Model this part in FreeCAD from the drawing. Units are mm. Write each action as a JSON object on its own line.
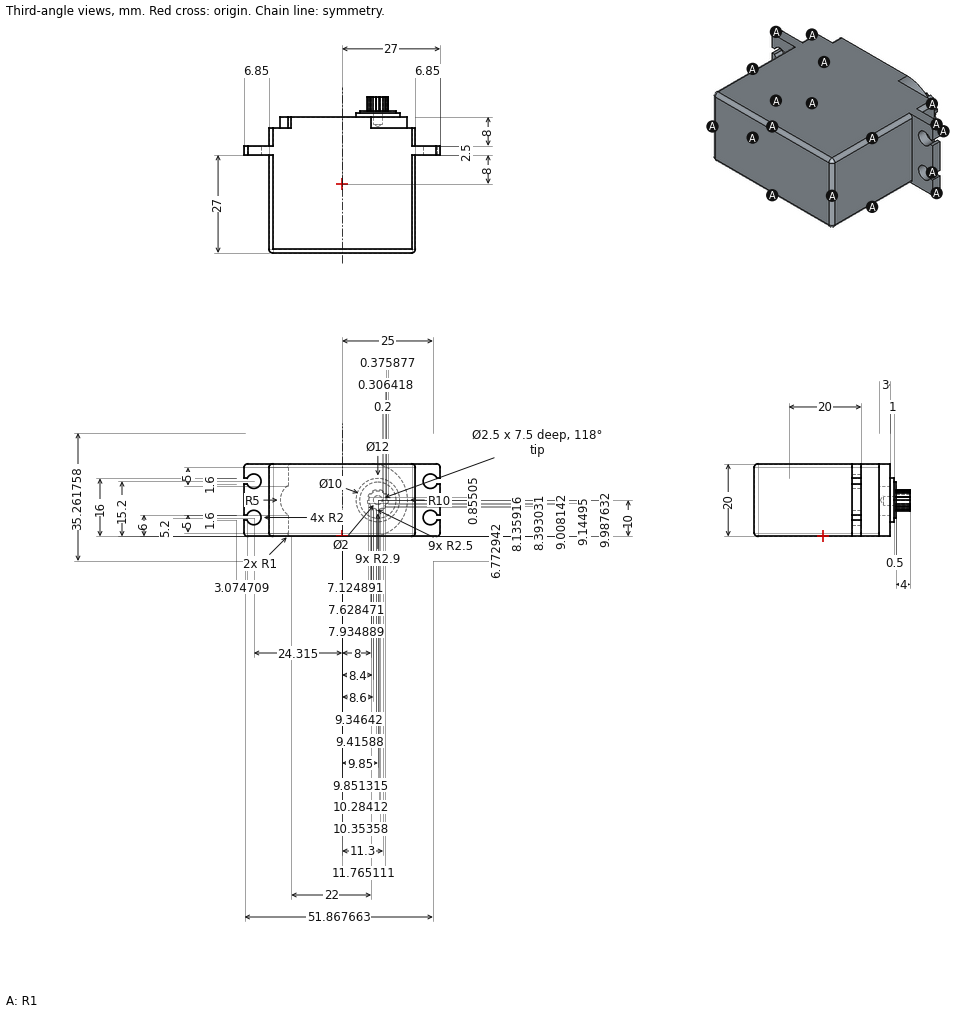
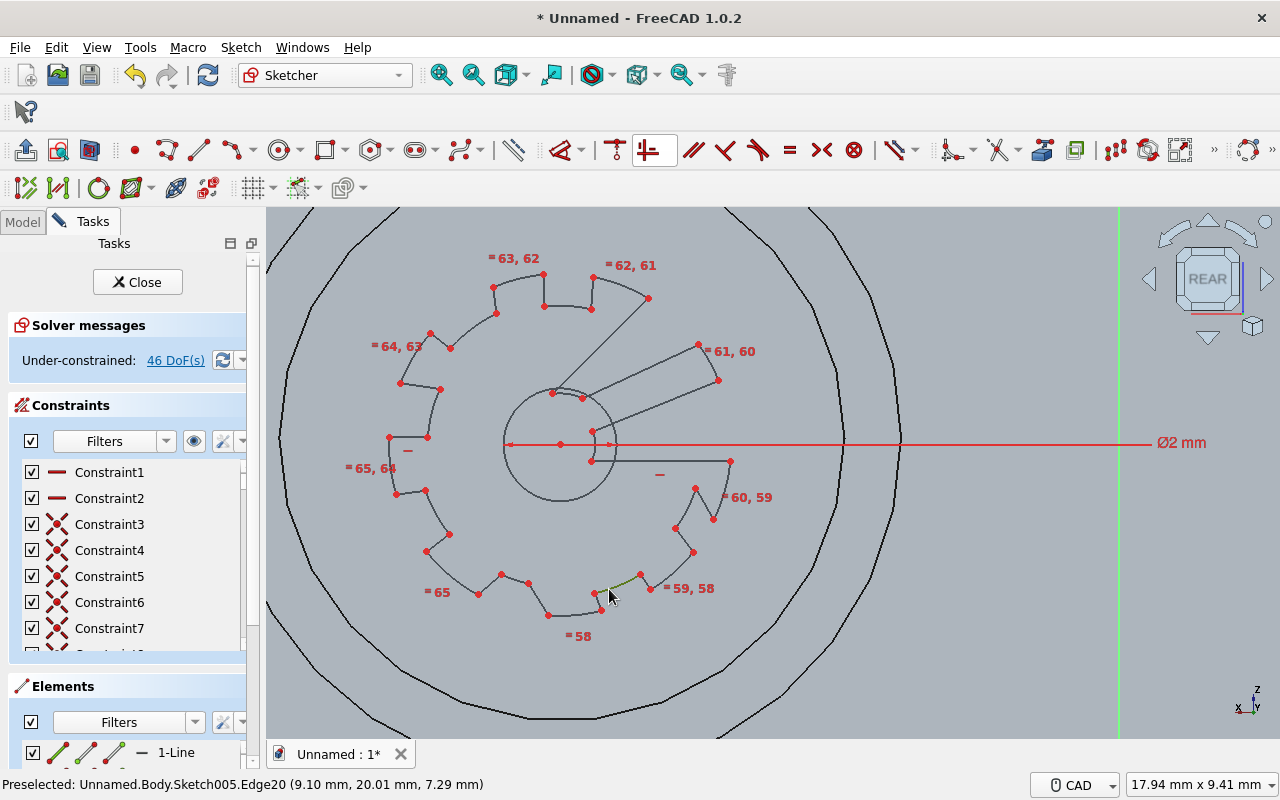
{"action": "left_click", "coordinate": [683, 517]}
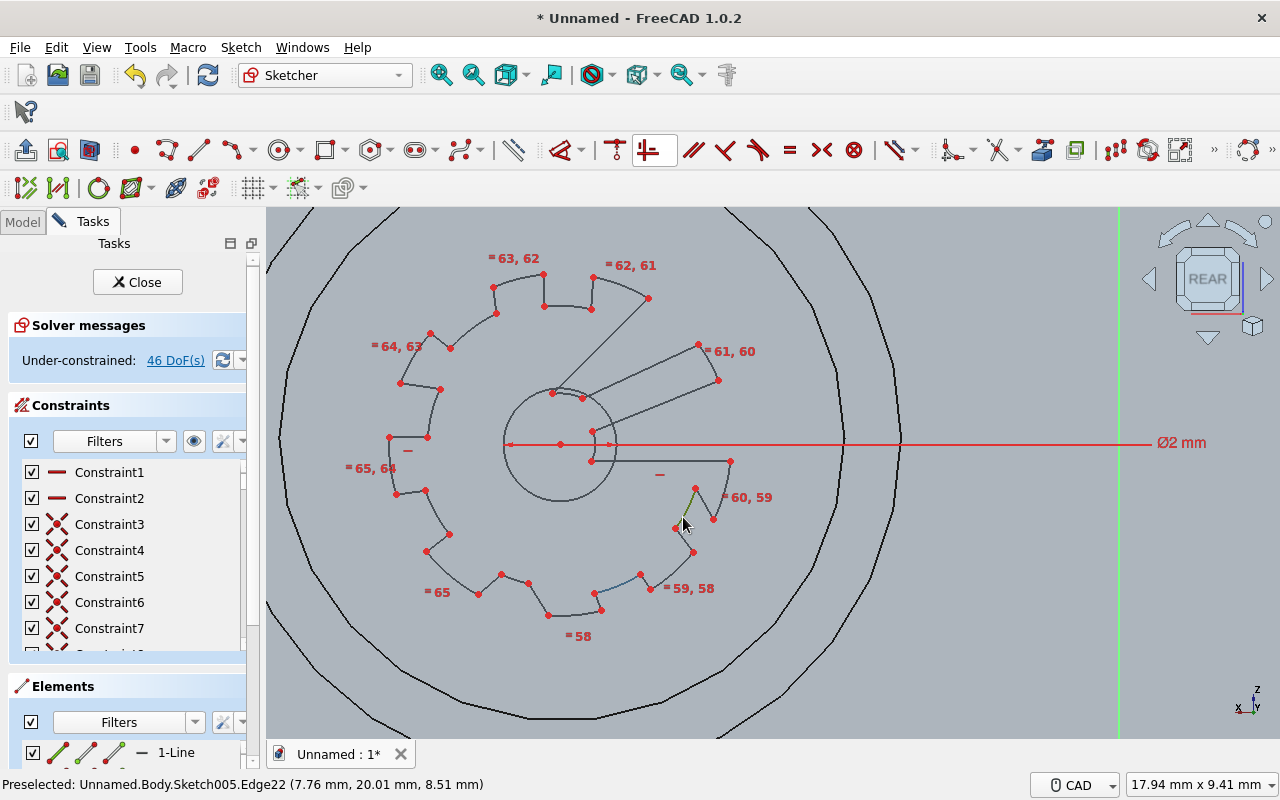
{"action": "scroll", "coordinate": [595, 440], "scroll_direction": "up", "scroll_amount": 3}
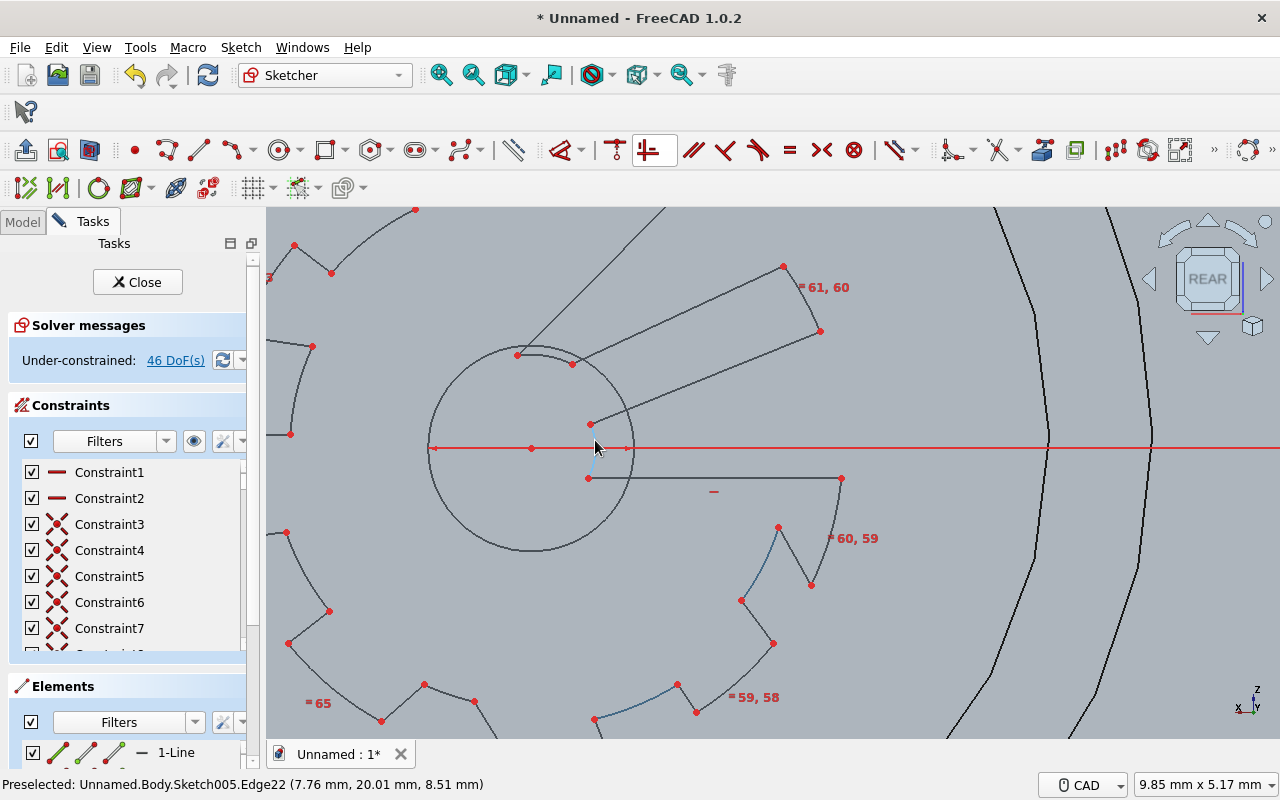
{"action": "left_click", "coordinate": [595, 440]}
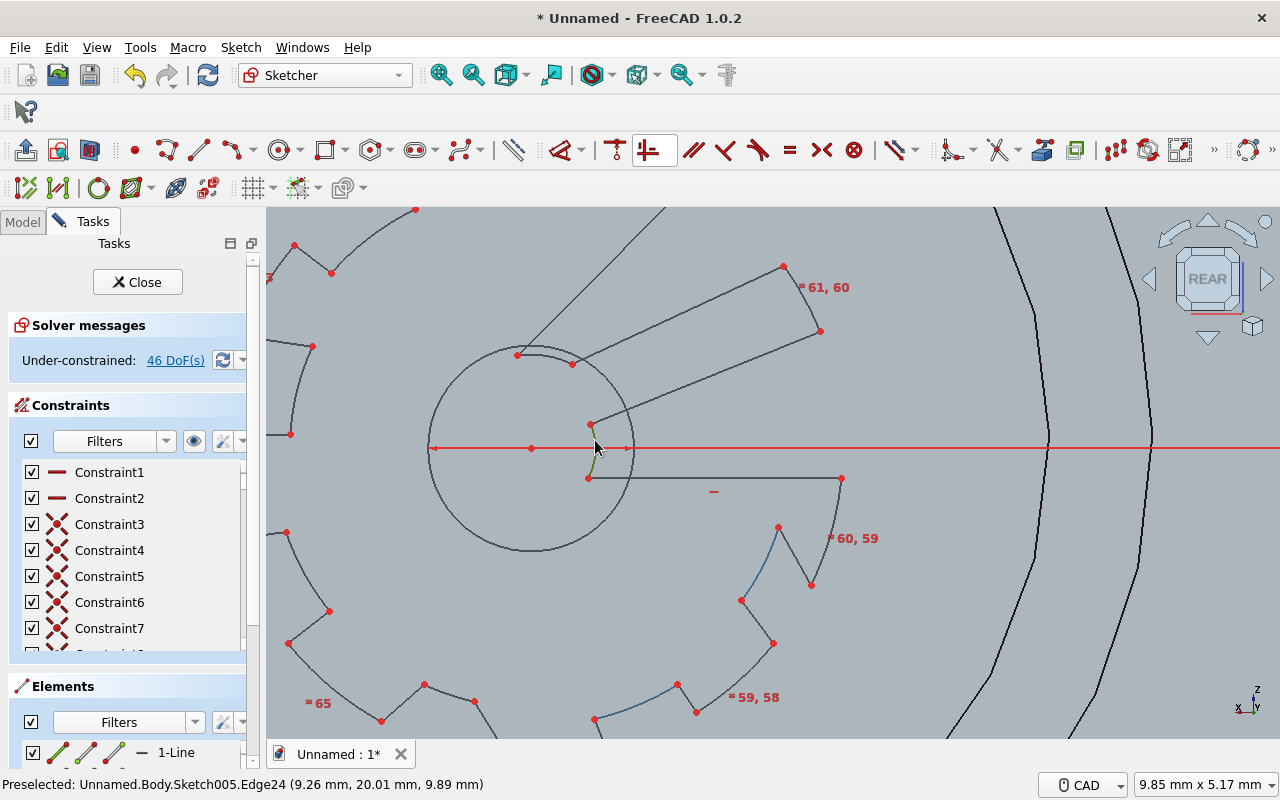
{"action": "scroll", "coordinate": [557, 358], "scroll_direction": "up", "scroll_amount": 2}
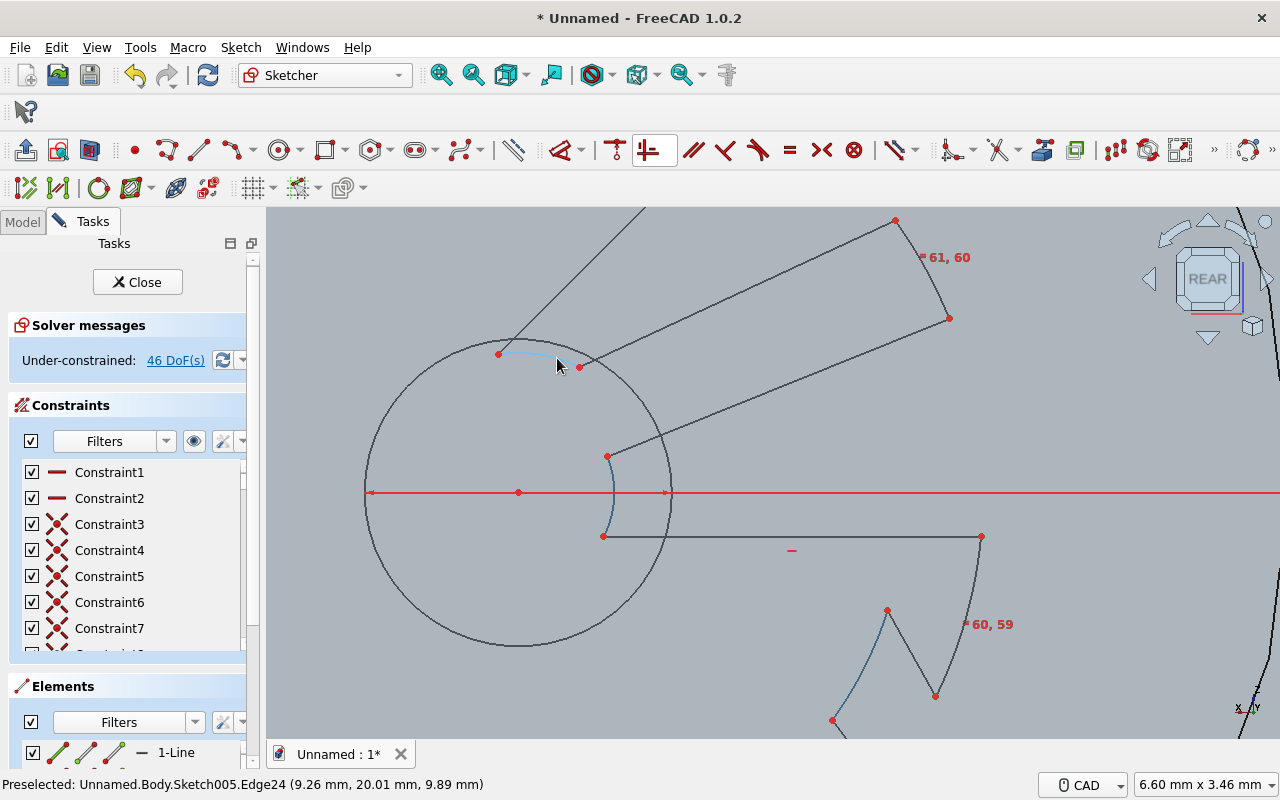
{"action": "left_click", "coordinate": [556, 358]}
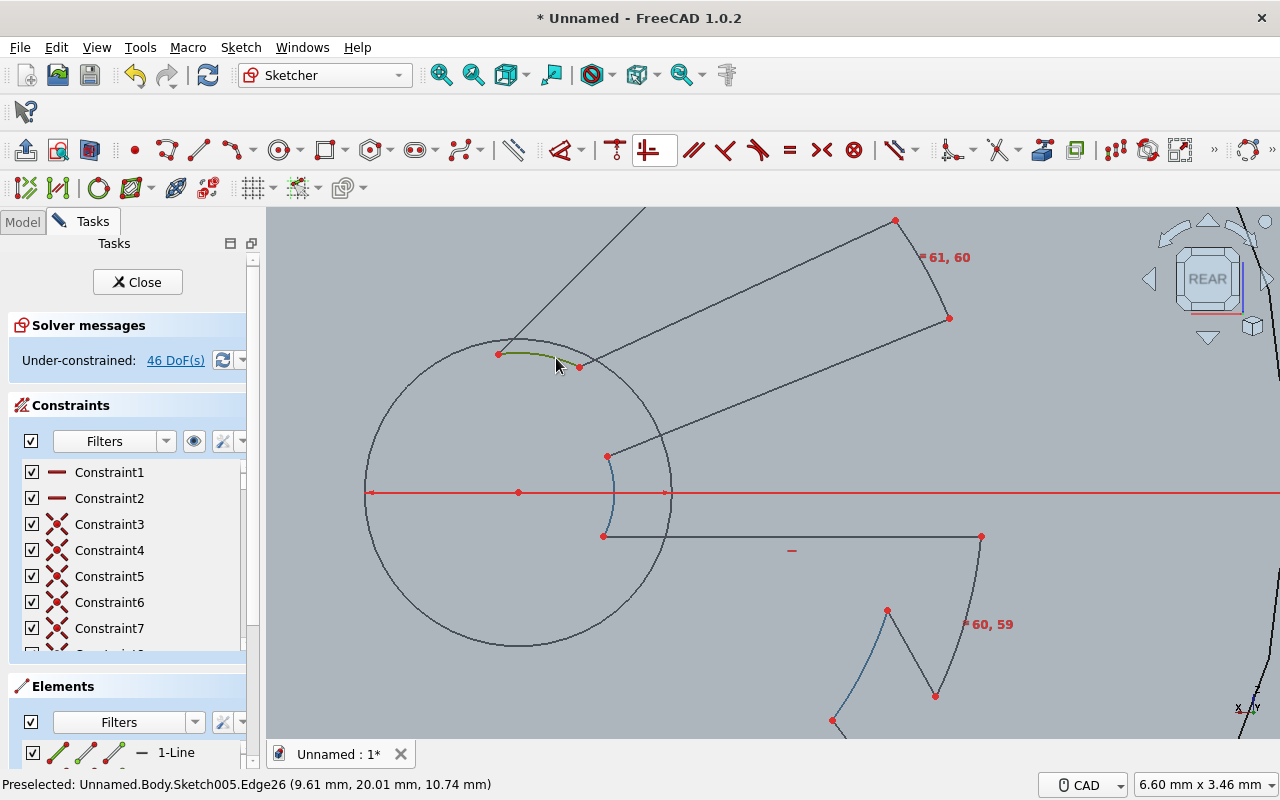
{"action": "scroll", "coordinate": [635, 364], "scroll_direction": "down", "scroll_amount": 9}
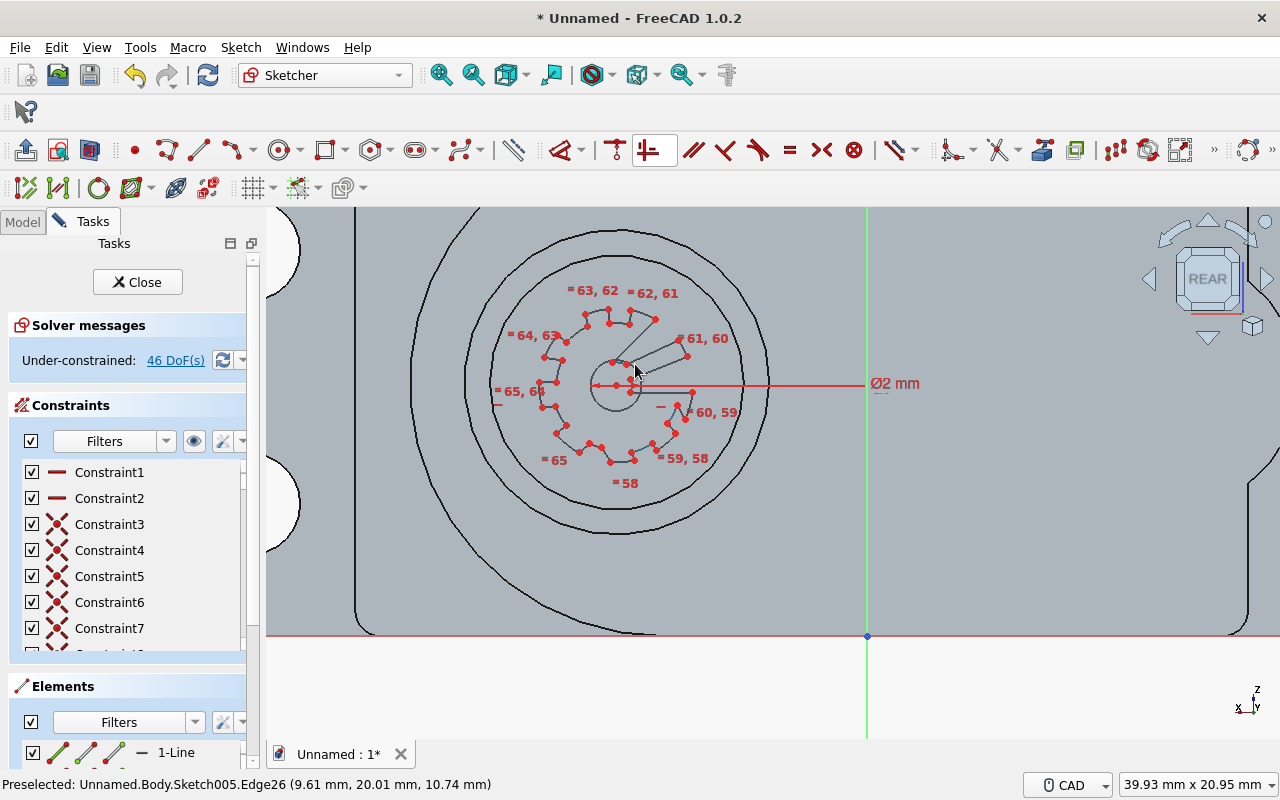
{"action": "scroll", "coordinate": [624, 324], "scroll_direction": "up", "scroll_amount": 4}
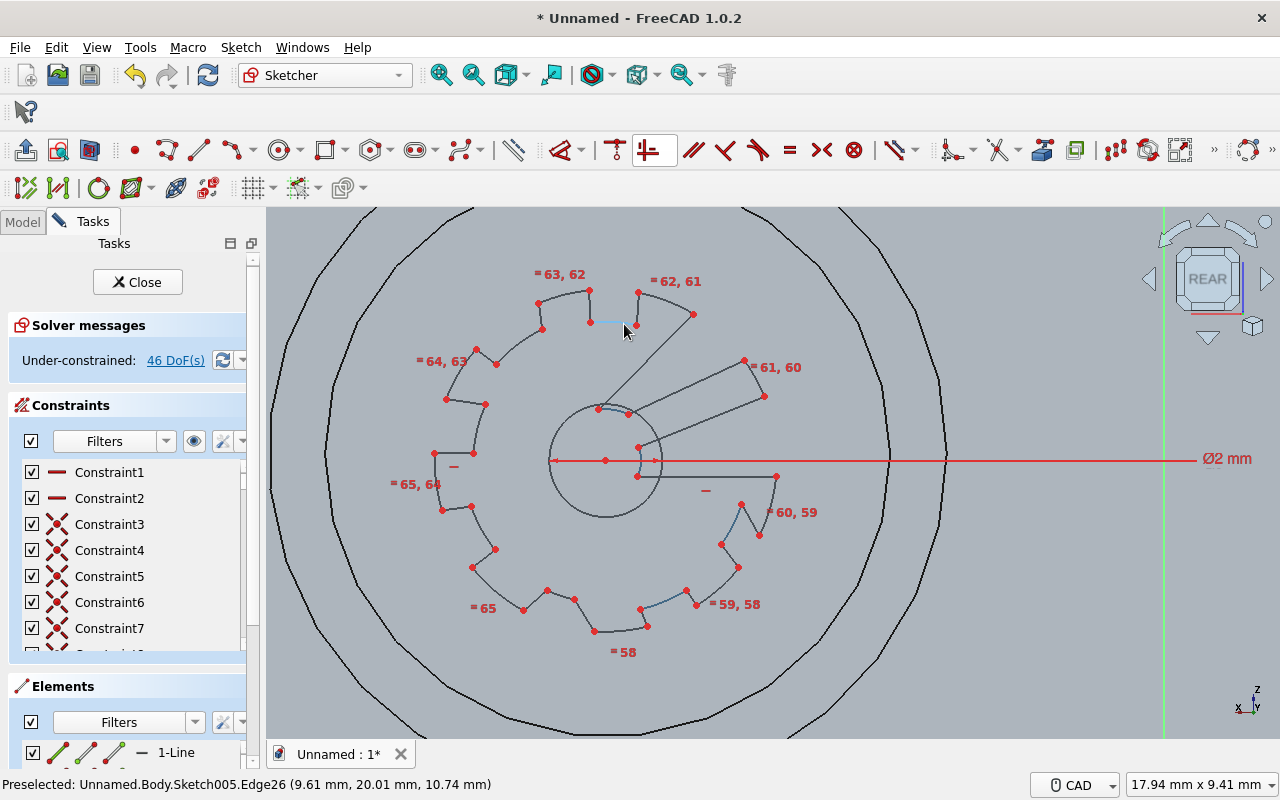
{"action": "left_click", "coordinate": [623, 323]}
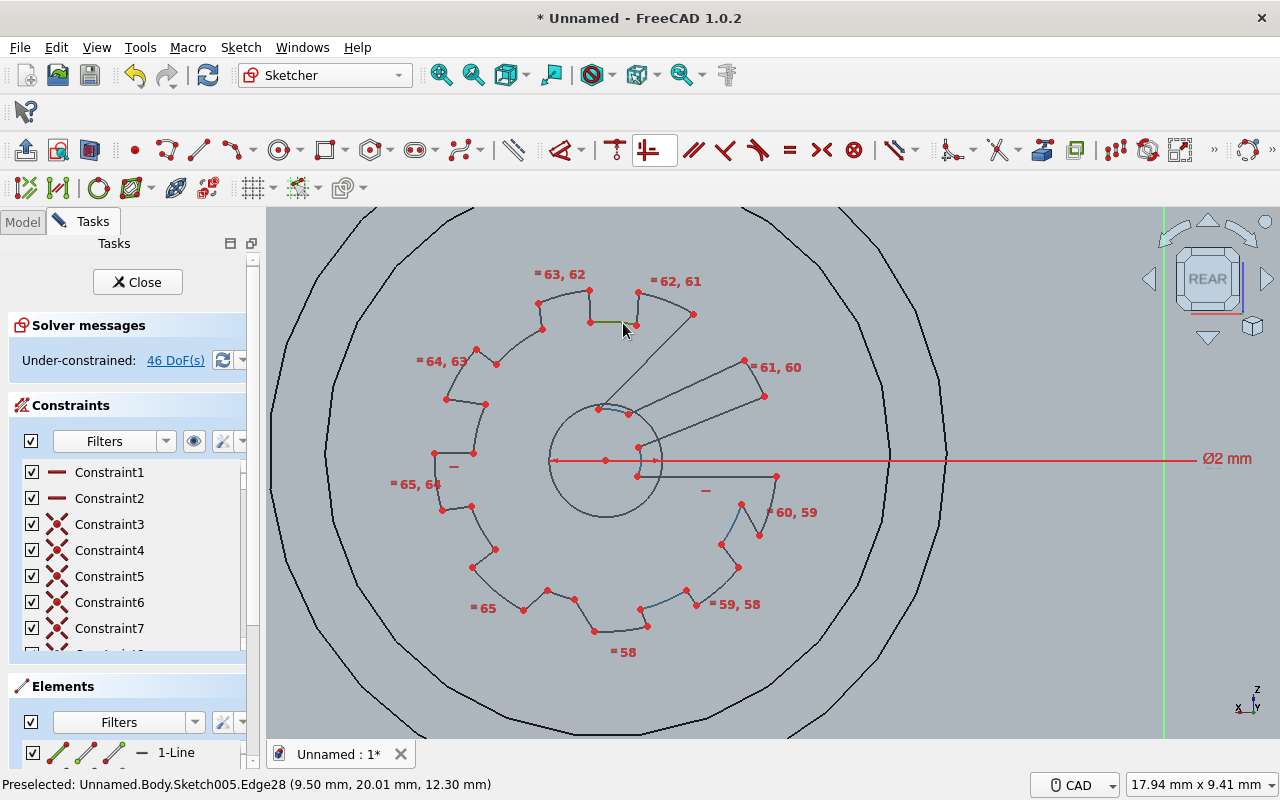
{"action": "left_click", "coordinate": [527, 338]}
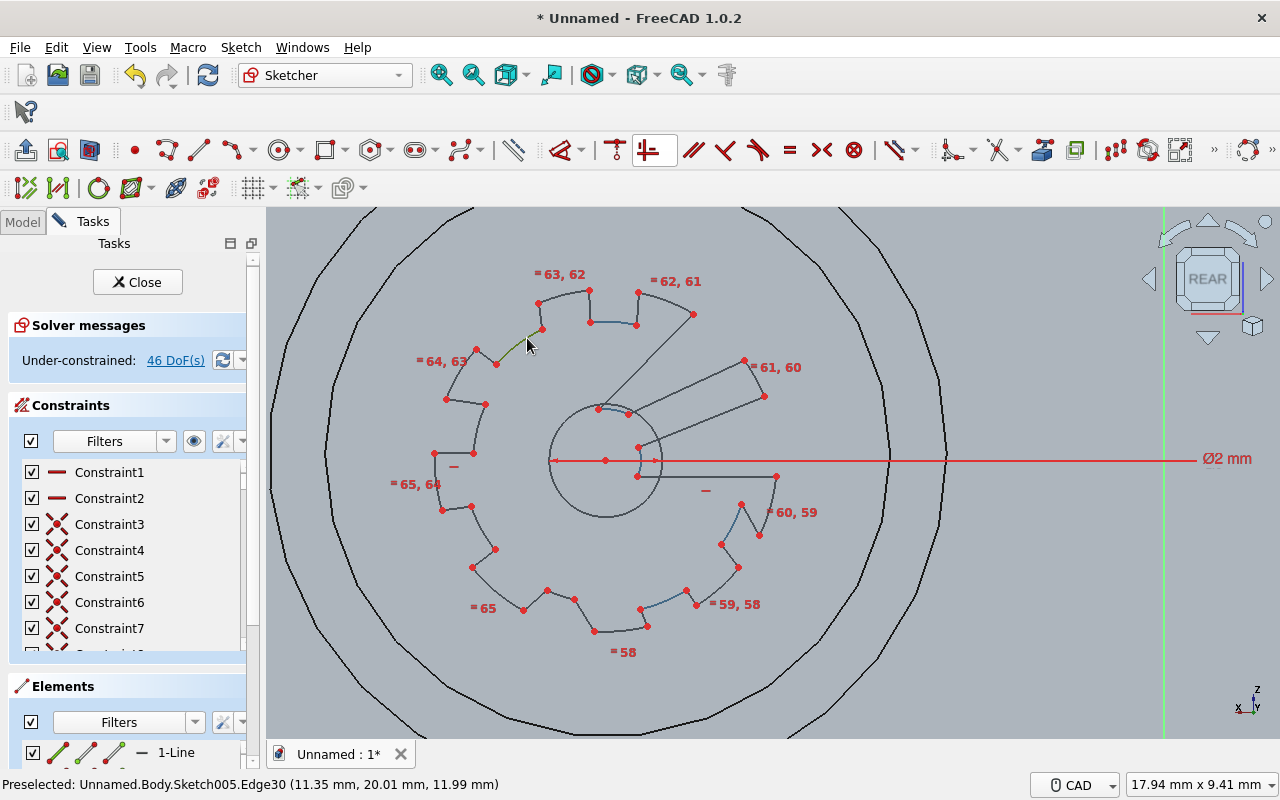
{"action": "left_click", "coordinate": [480, 419]}